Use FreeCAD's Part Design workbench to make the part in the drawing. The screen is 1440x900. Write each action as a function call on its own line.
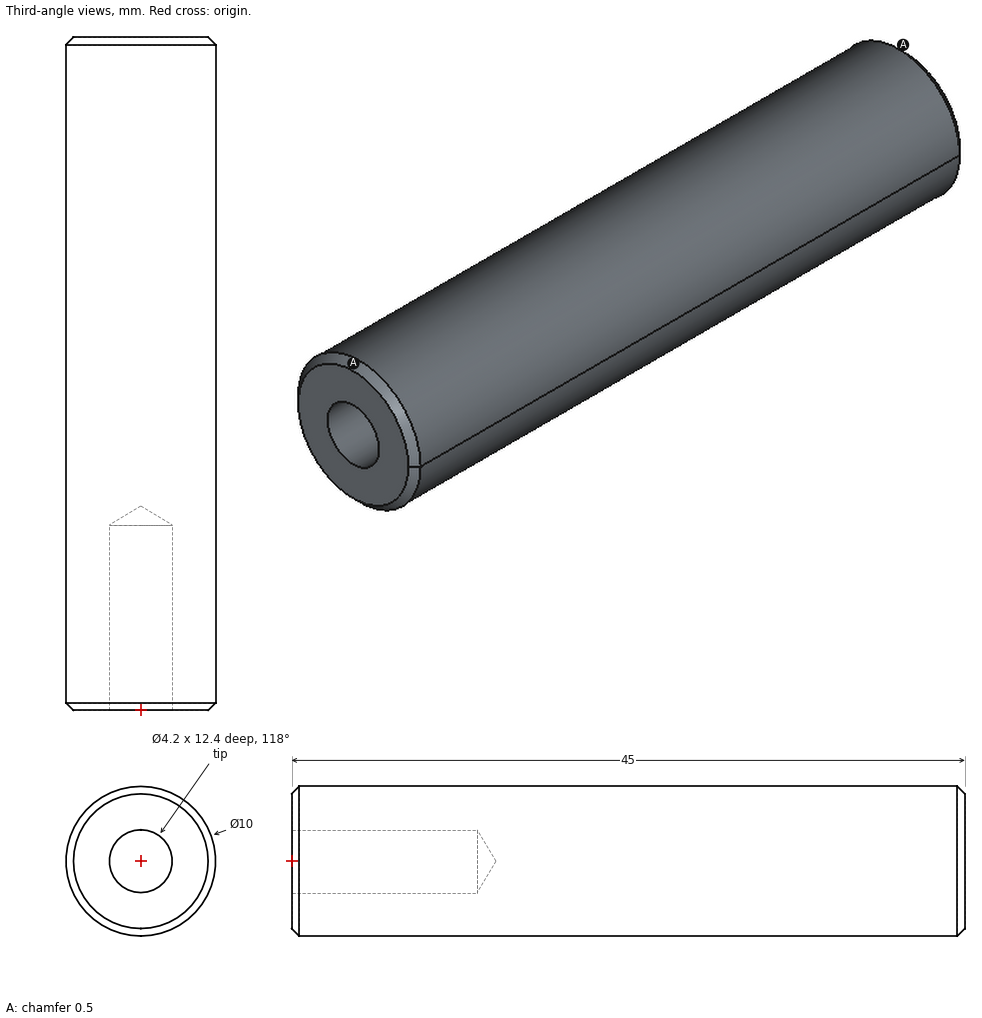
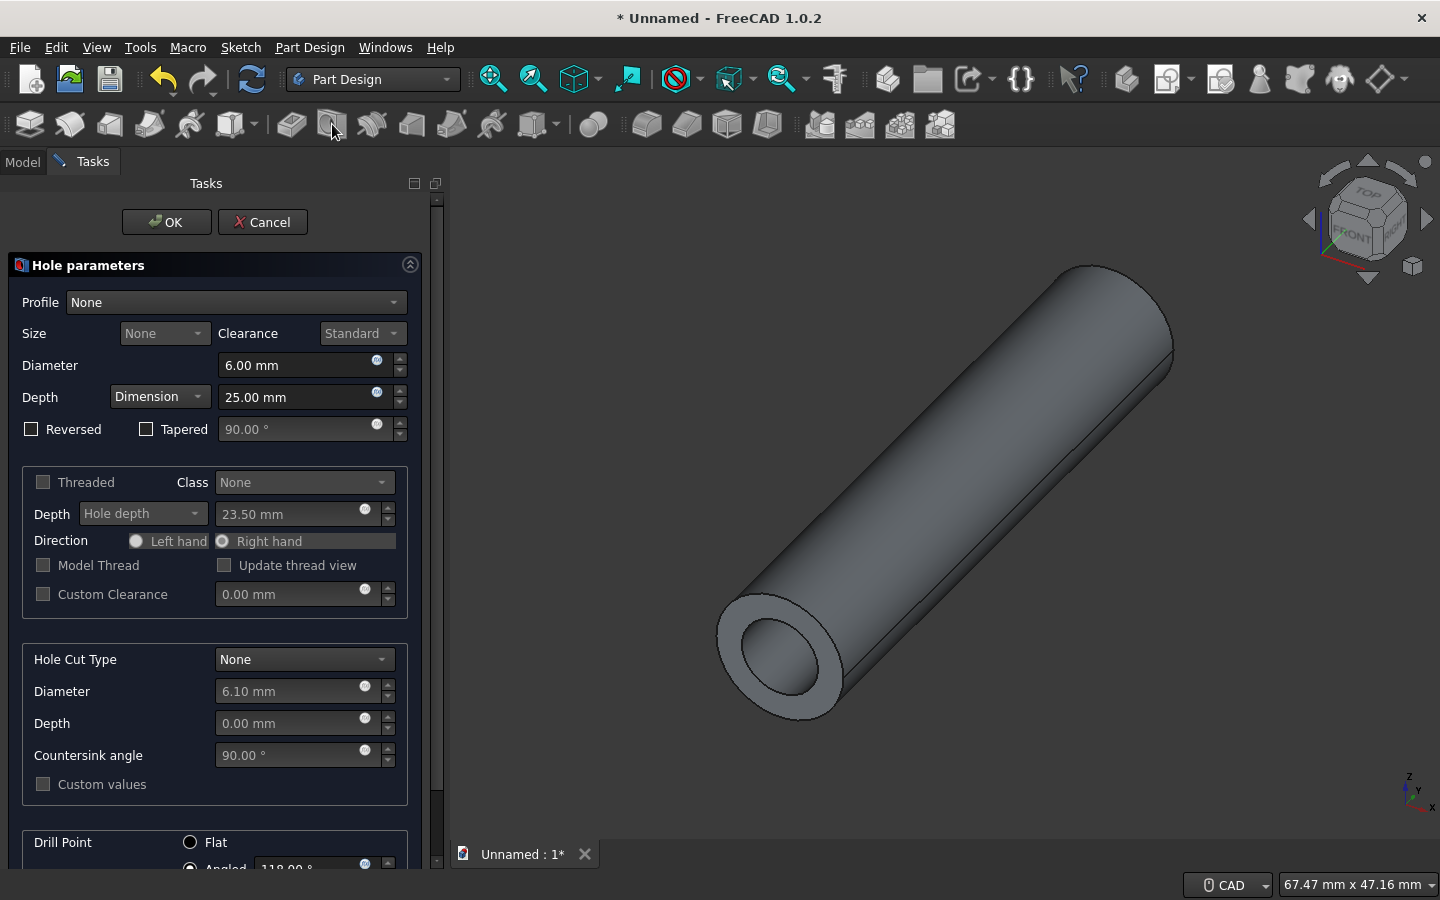
triple_click(305, 365)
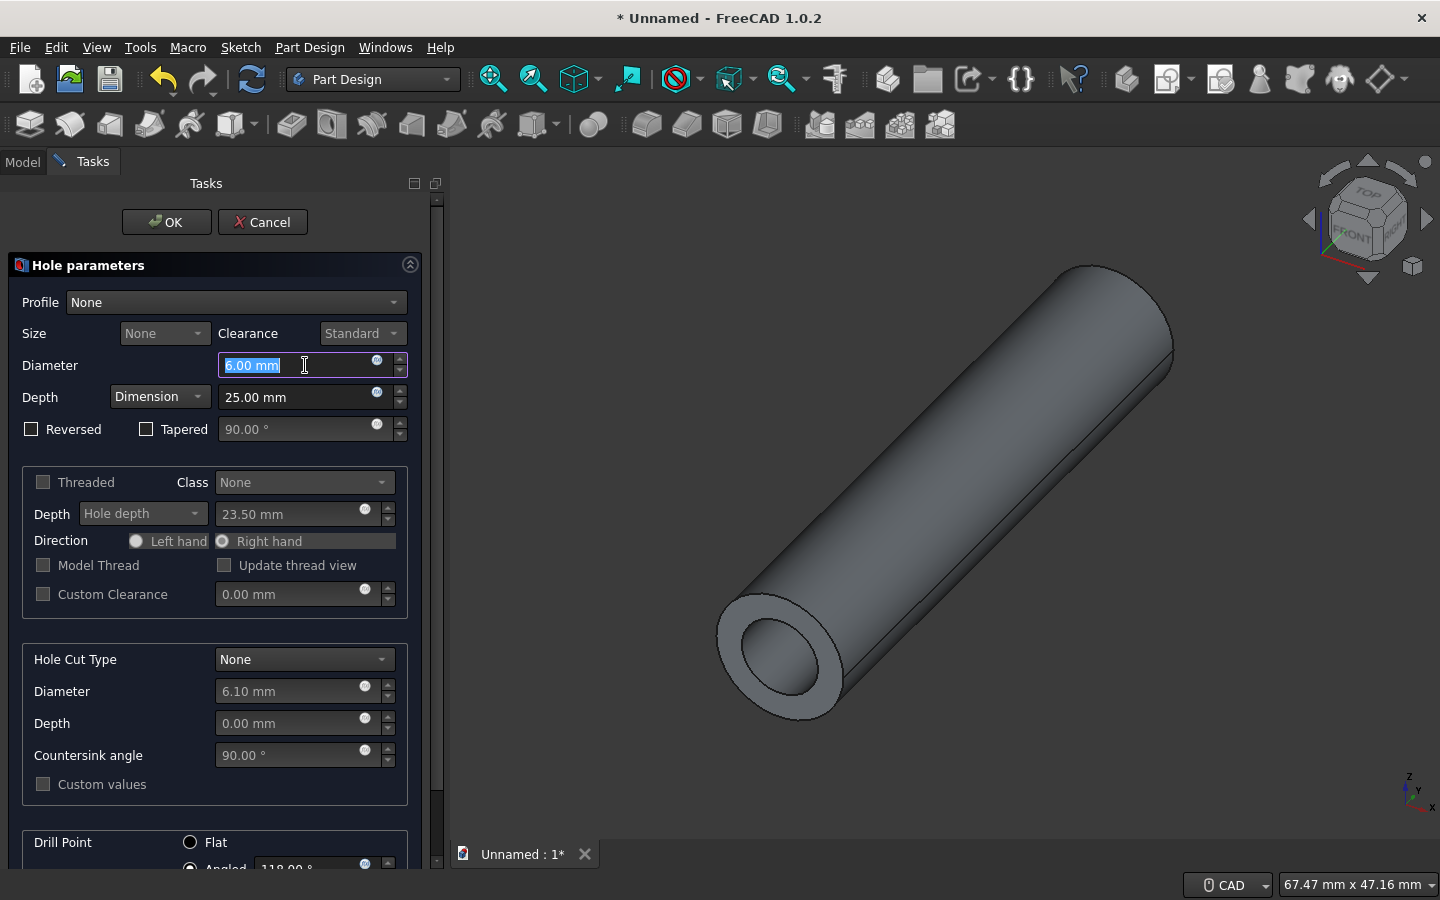
text(4.2)
key(Tab)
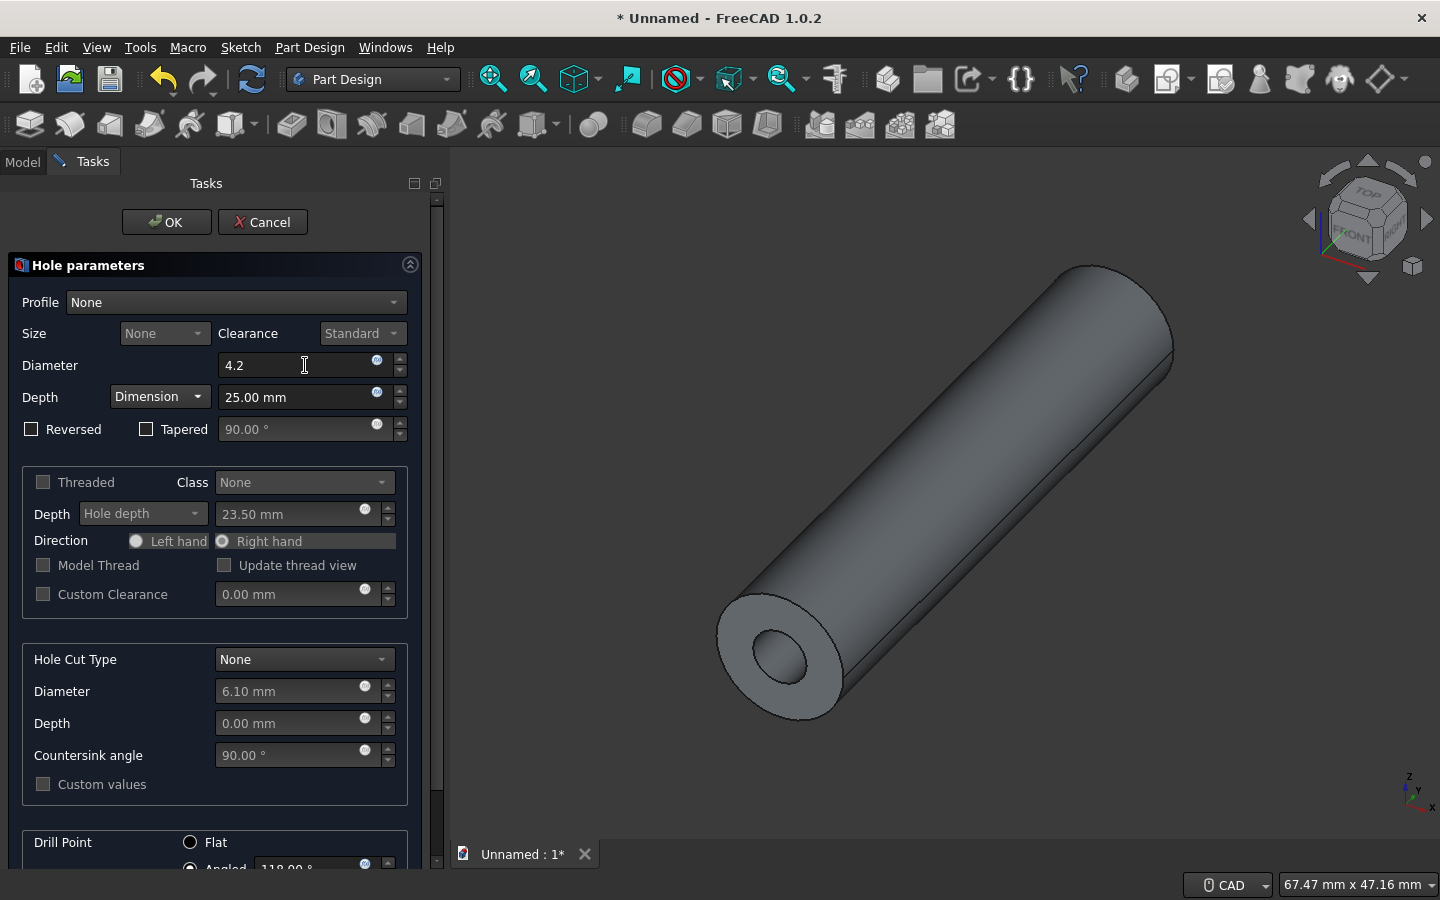
triple_click(305, 397)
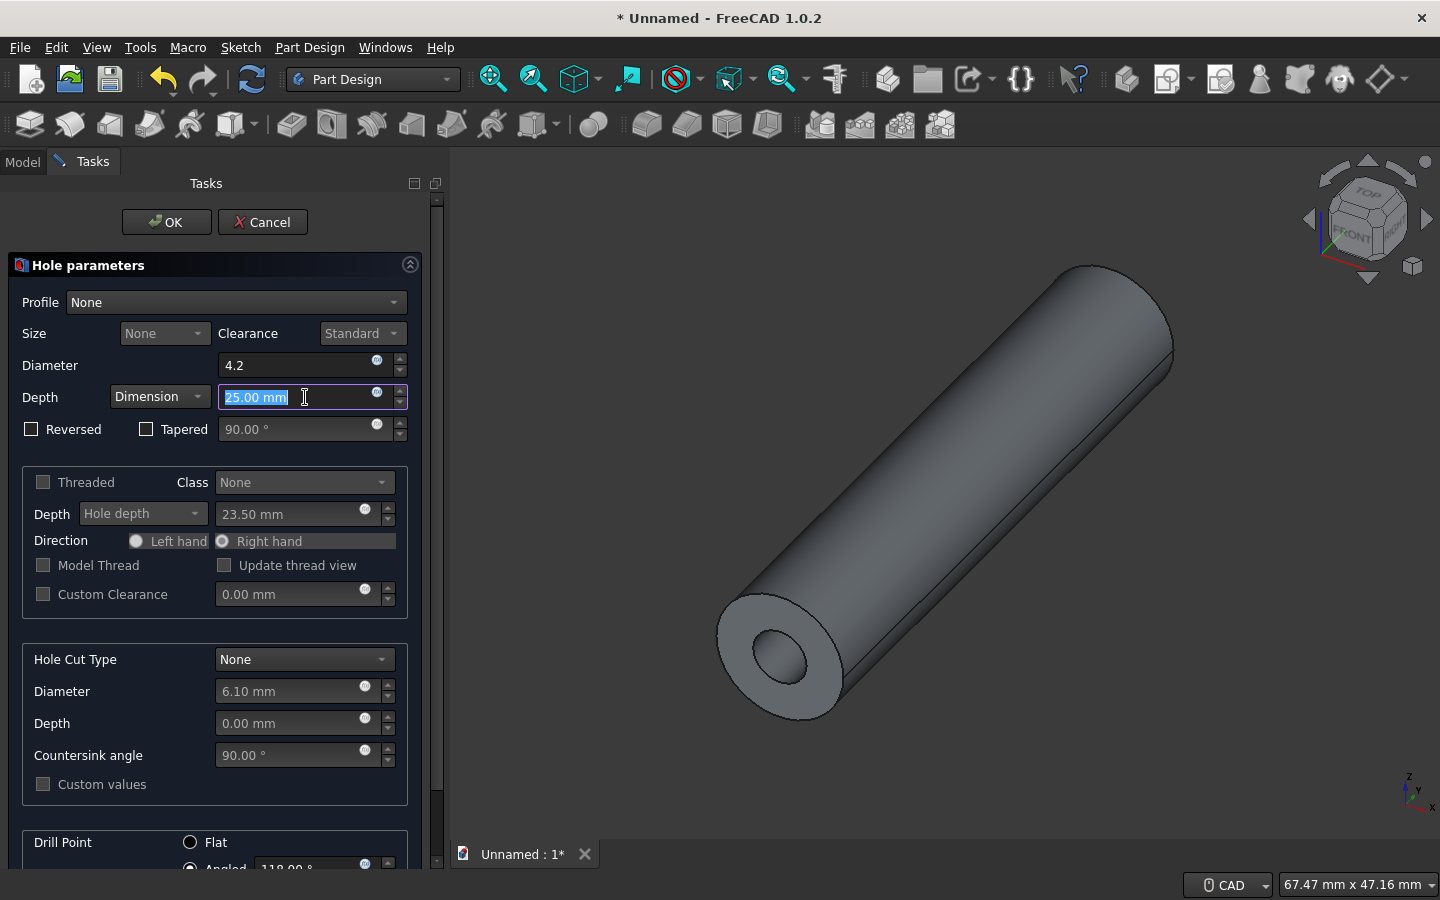
text(12.4)
key(Tab)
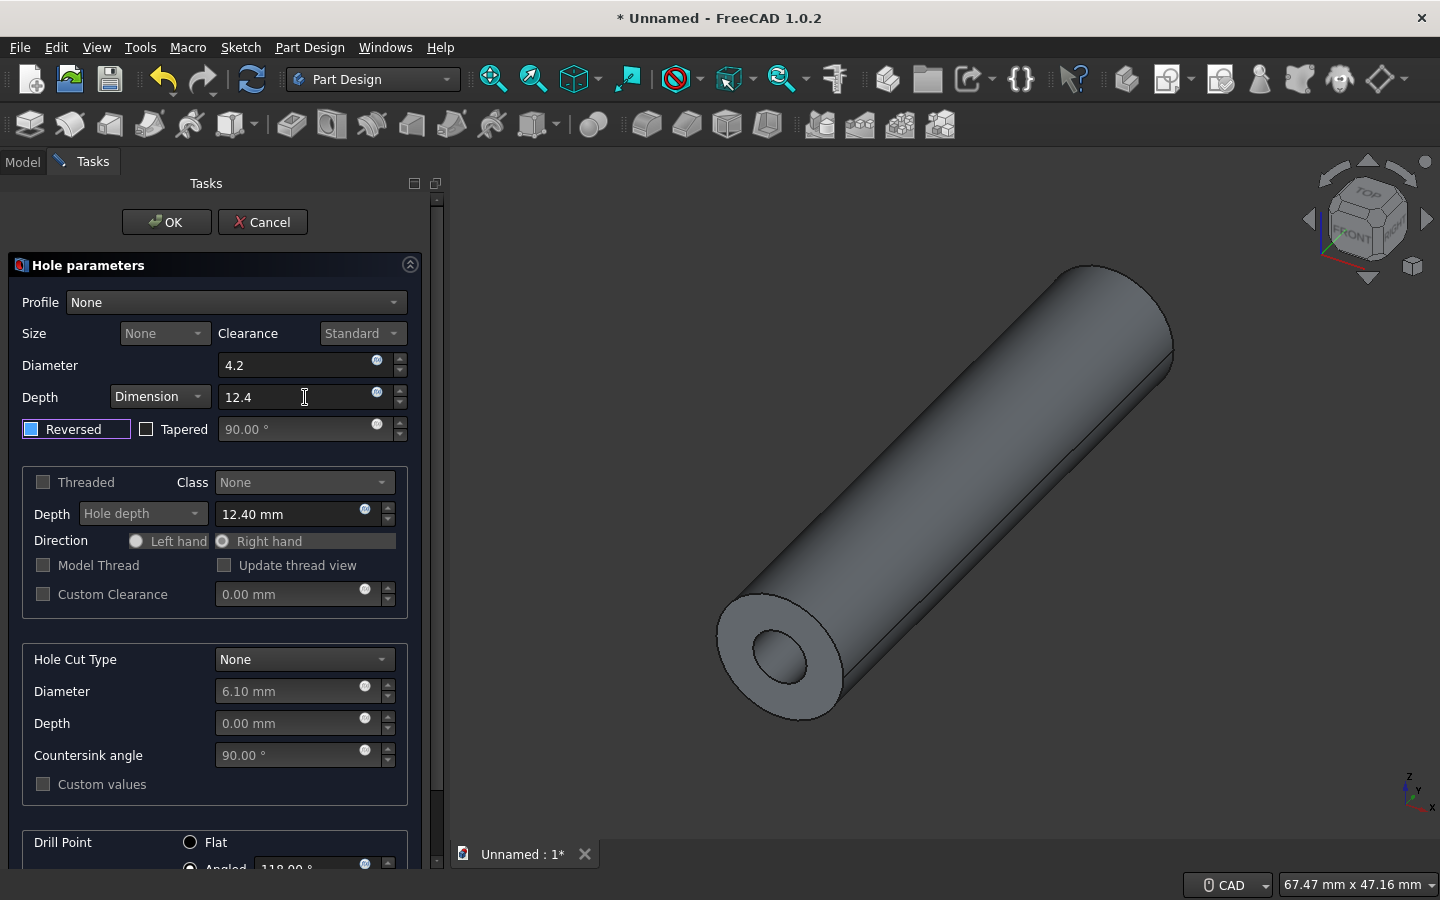
click(167, 222)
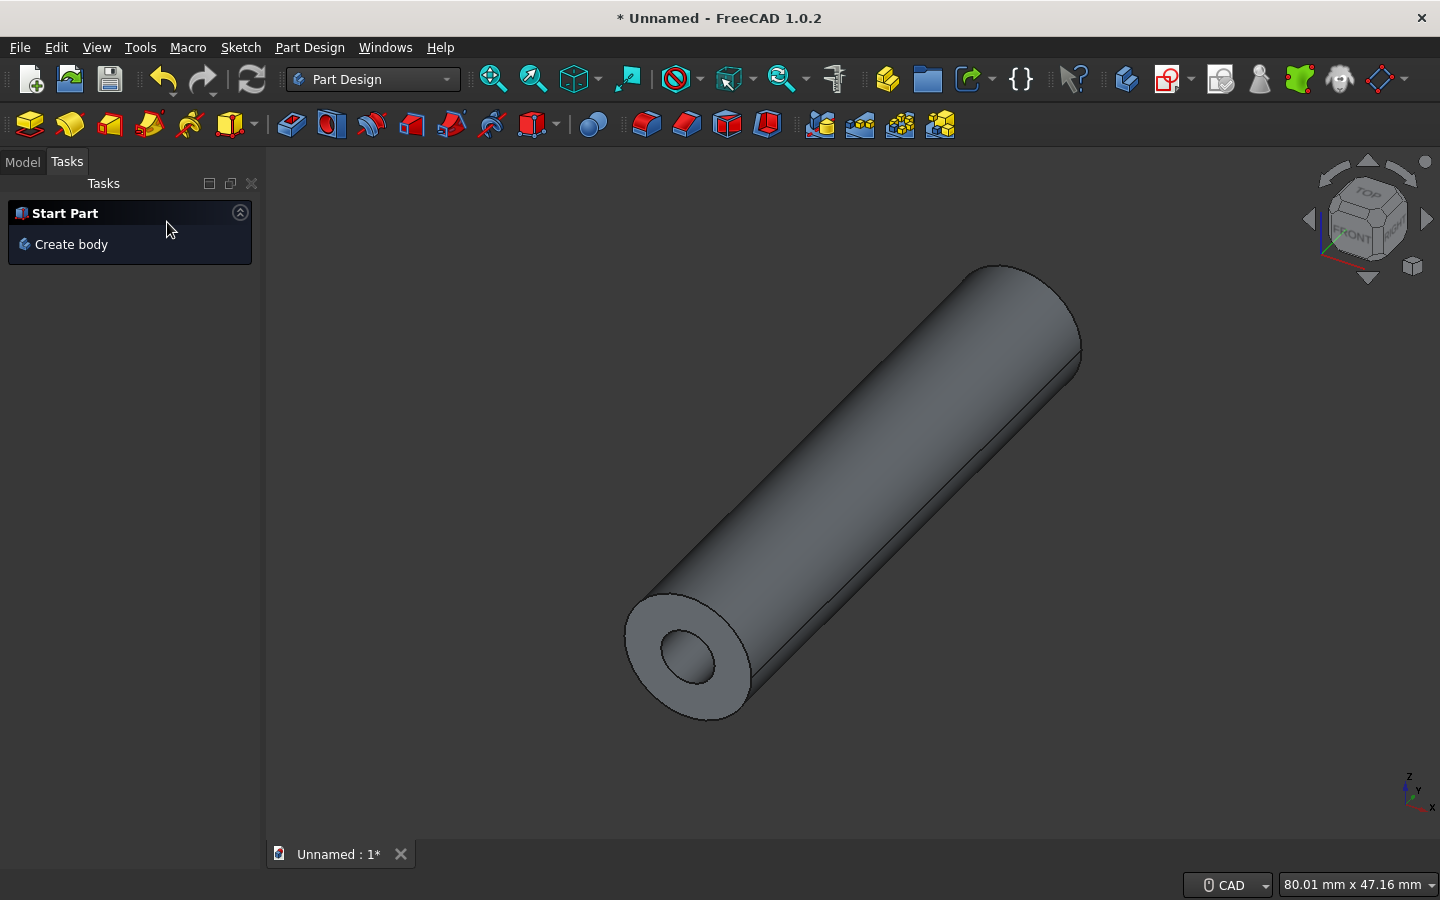
click(637, 604)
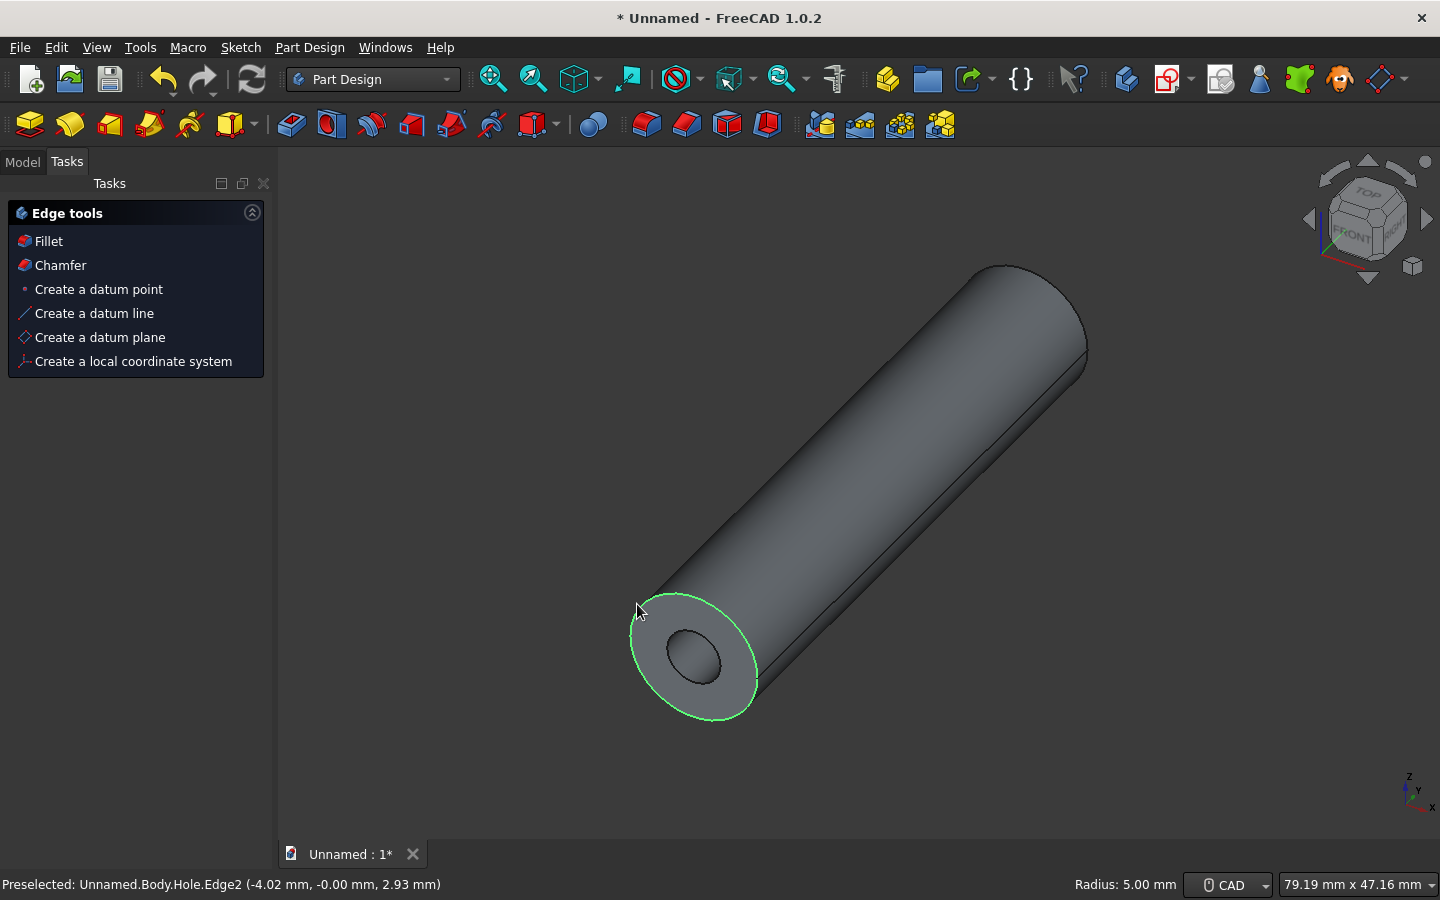
click(1004, 264, ctrl)